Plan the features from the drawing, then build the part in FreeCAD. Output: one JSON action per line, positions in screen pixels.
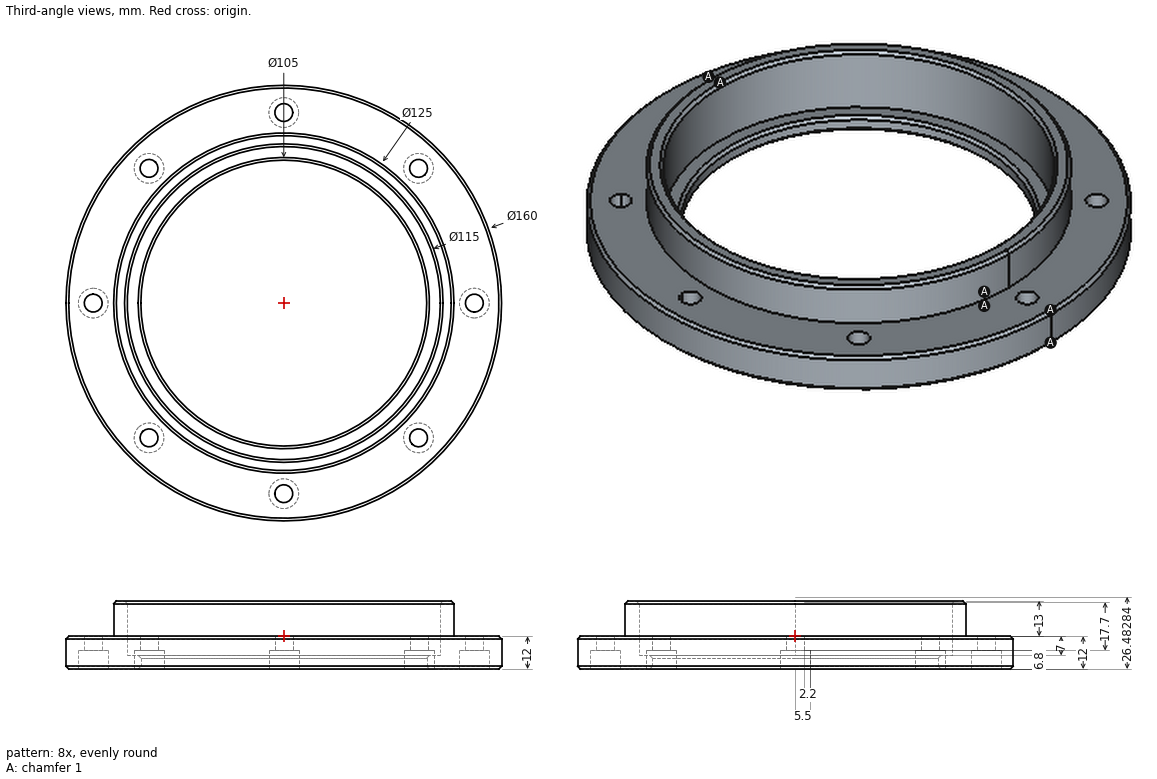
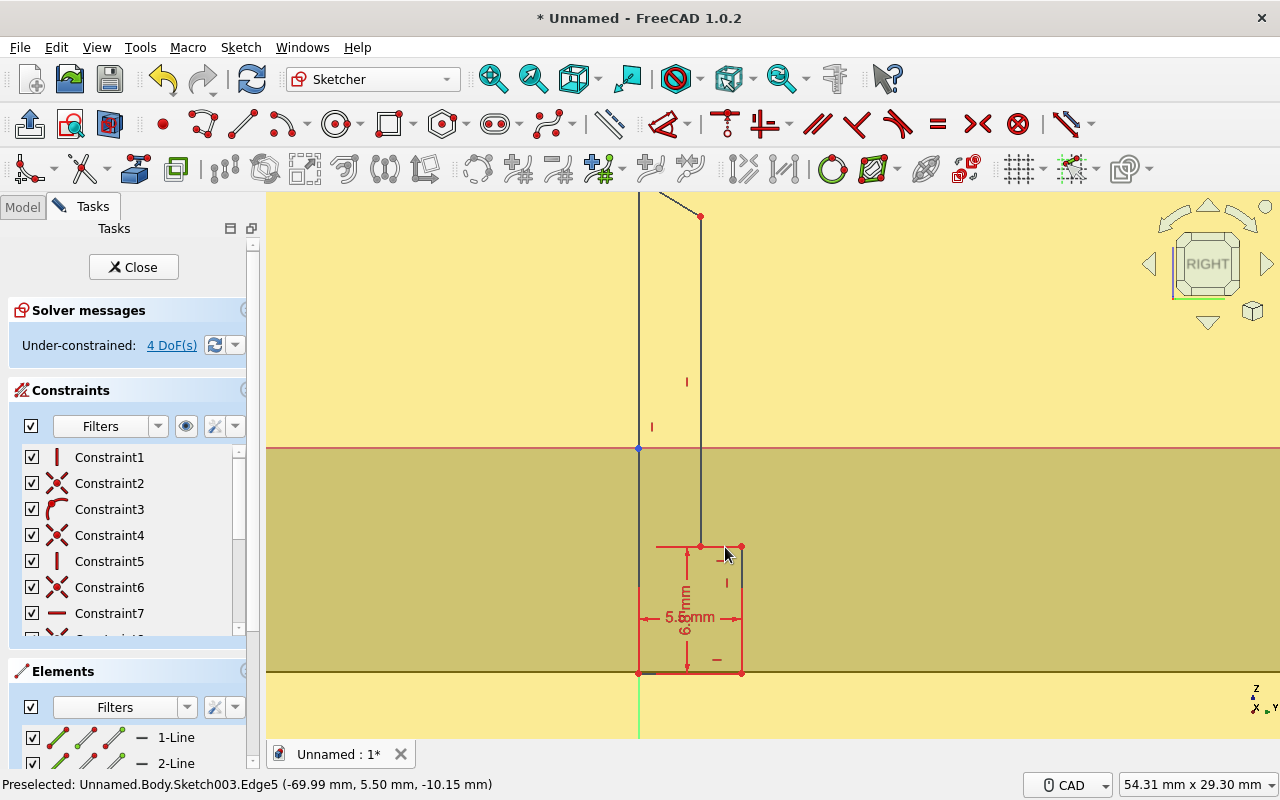
{"action": "left_click", "coordinate": [725, 547]}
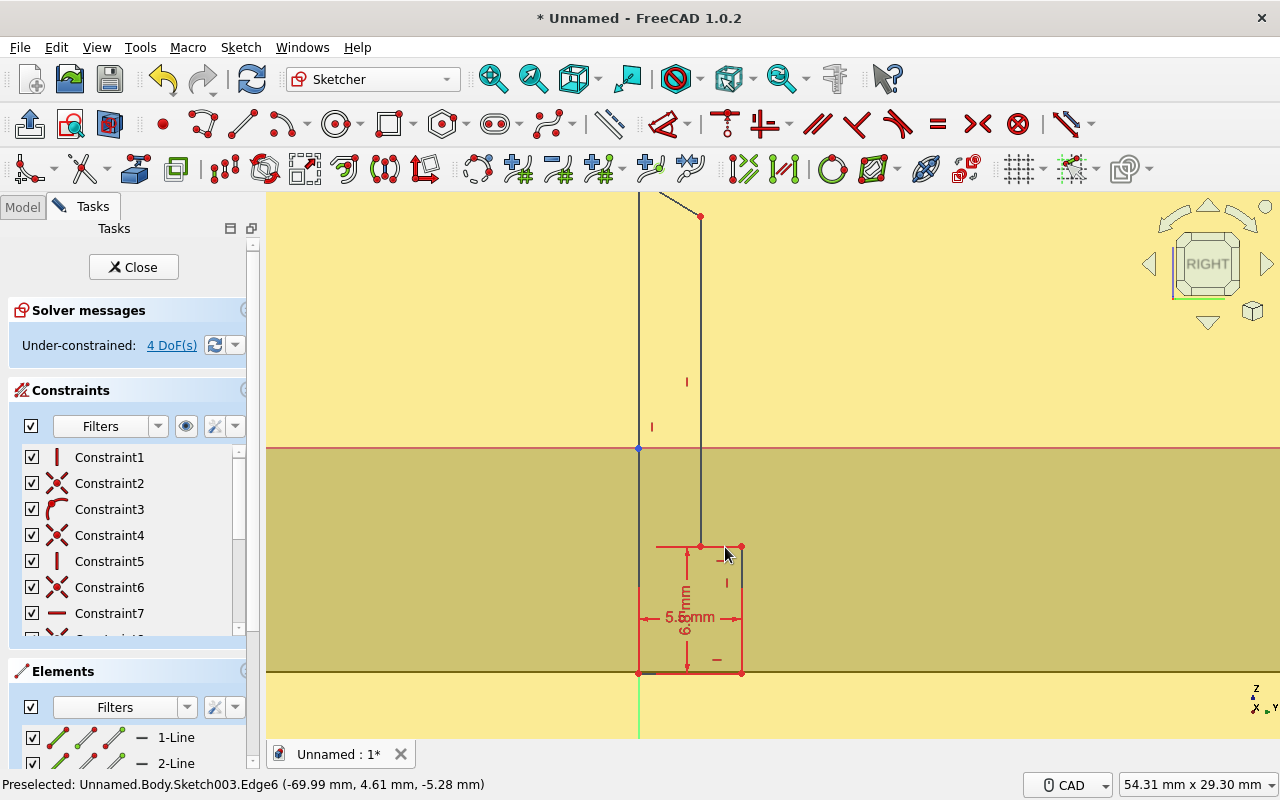
{"action": "key", "text": "l"}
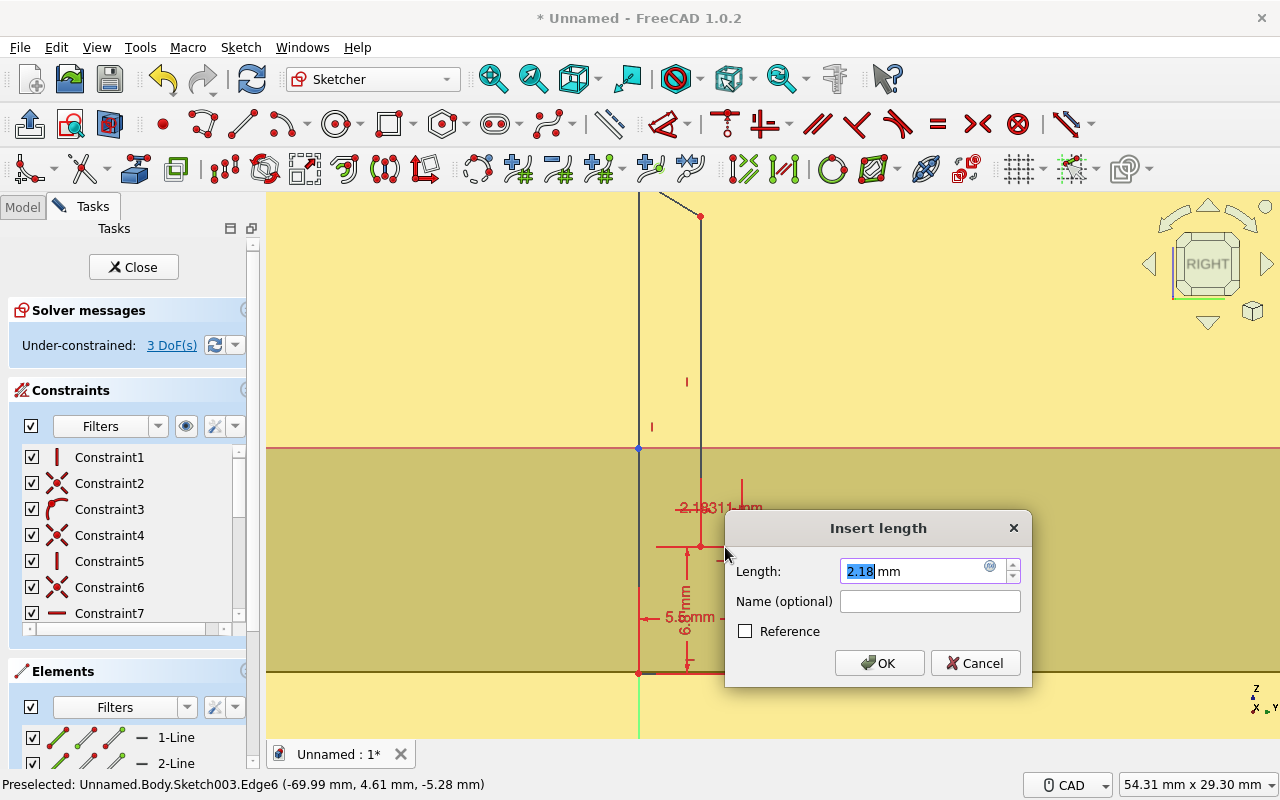
{"action": "type", "text": "2.2"}
{"action": "key", "text": "Return"}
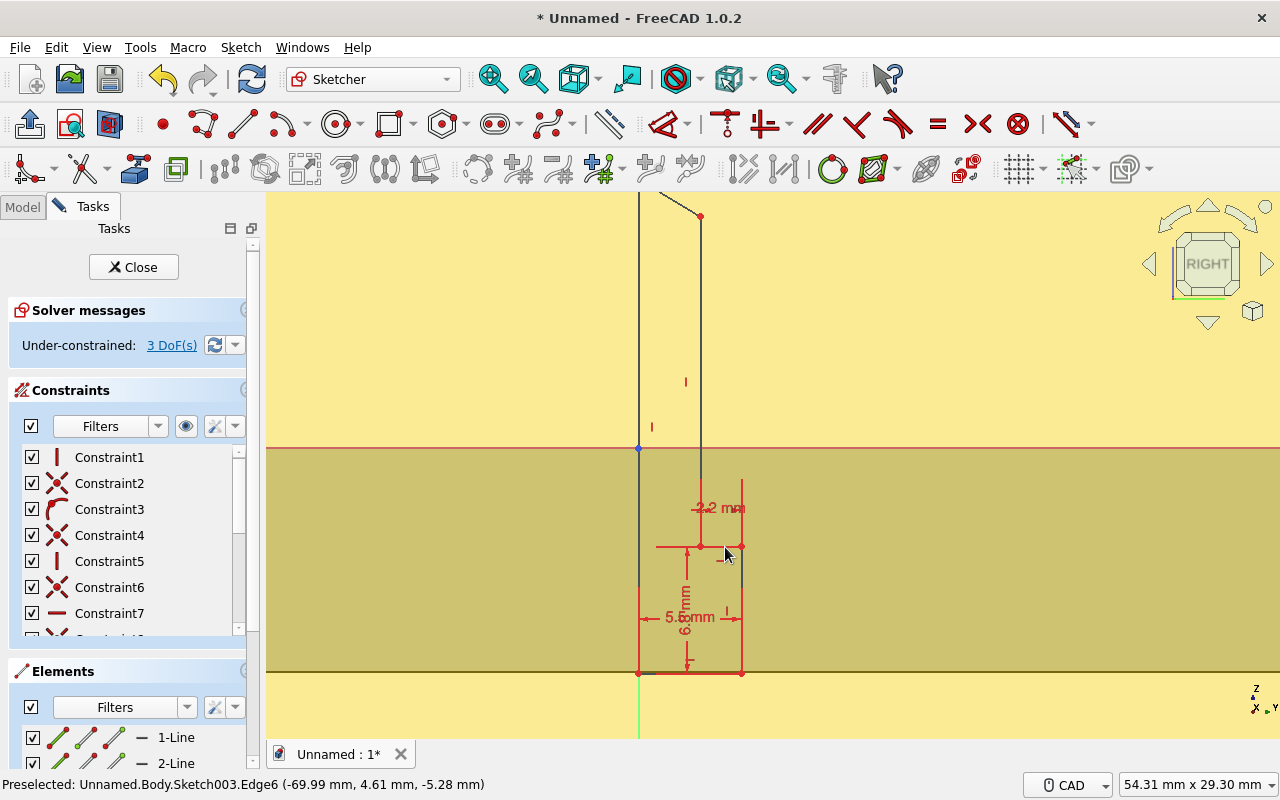
{"action": "left_click", "coordinate": [639, 674]}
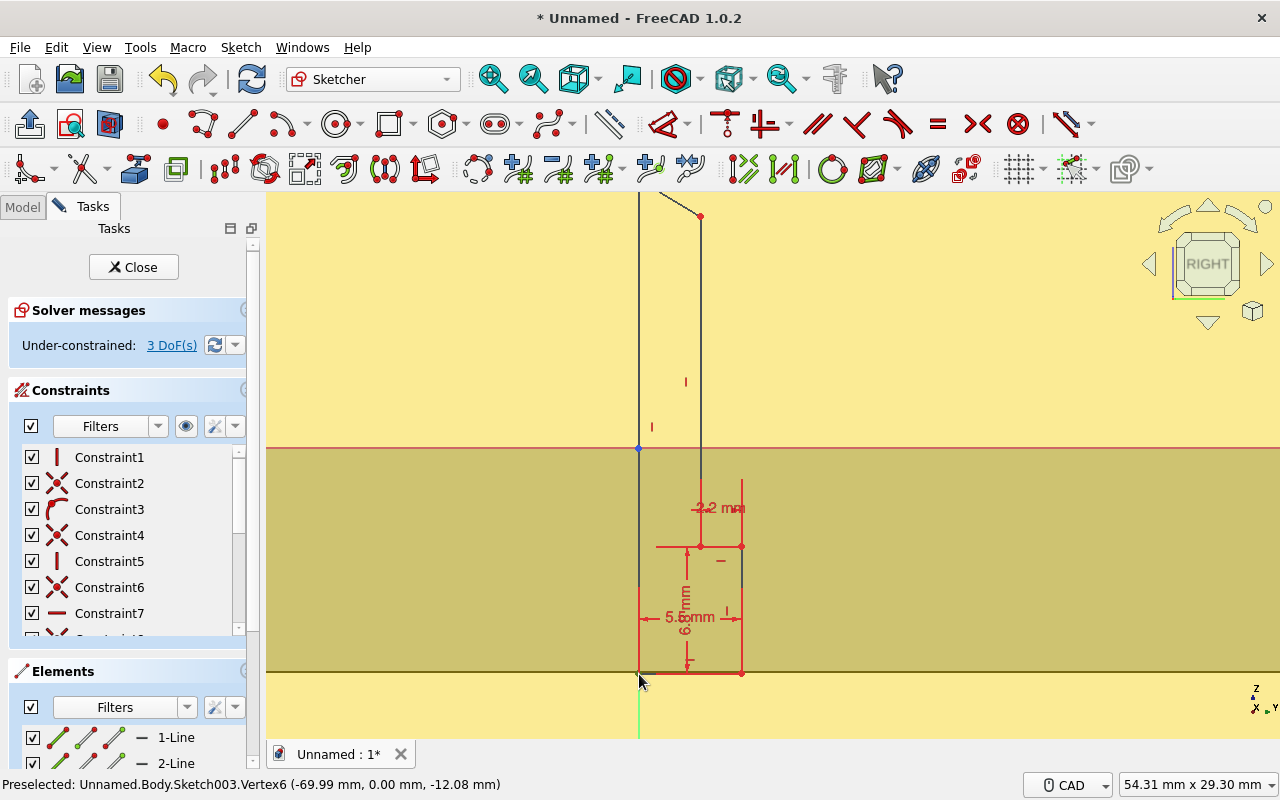
{"action": "key", "text": "i"}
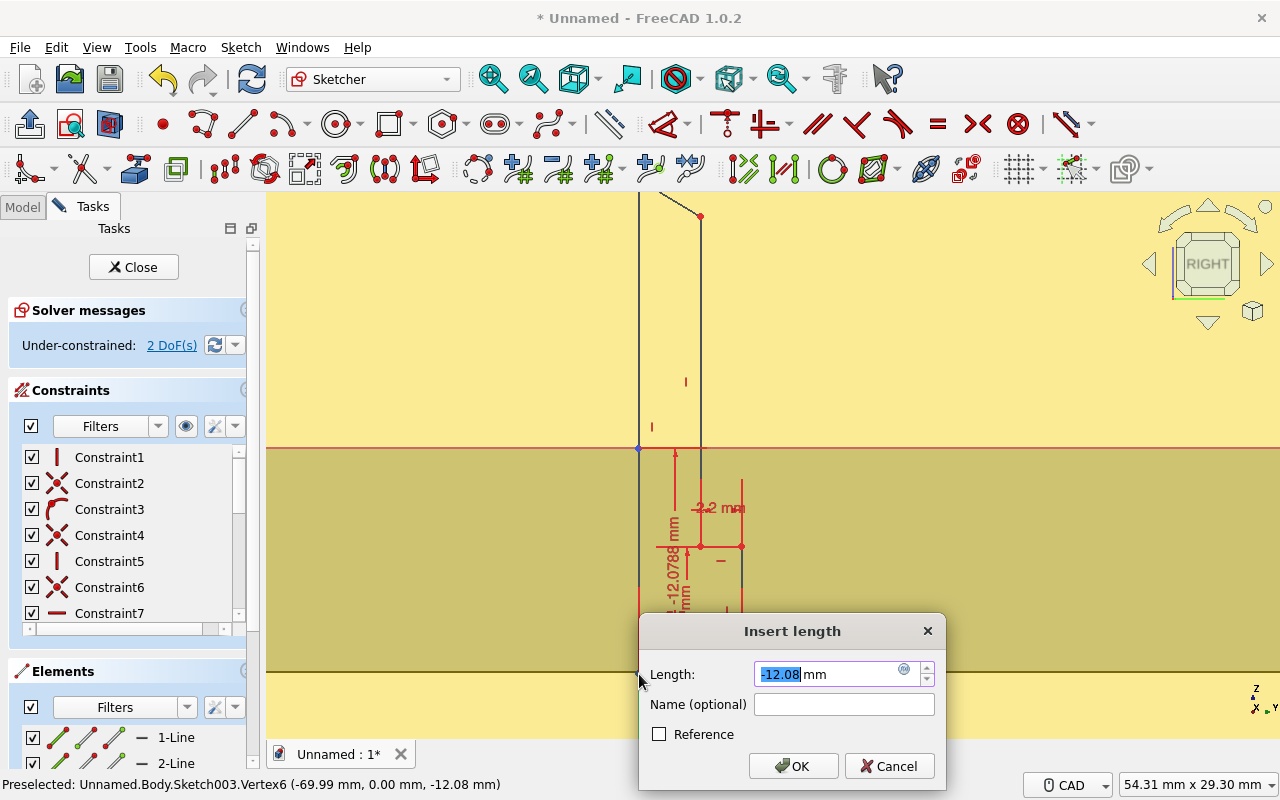
{"action": "type", "text": "-12"}
{"action": "key", "text": "Return"}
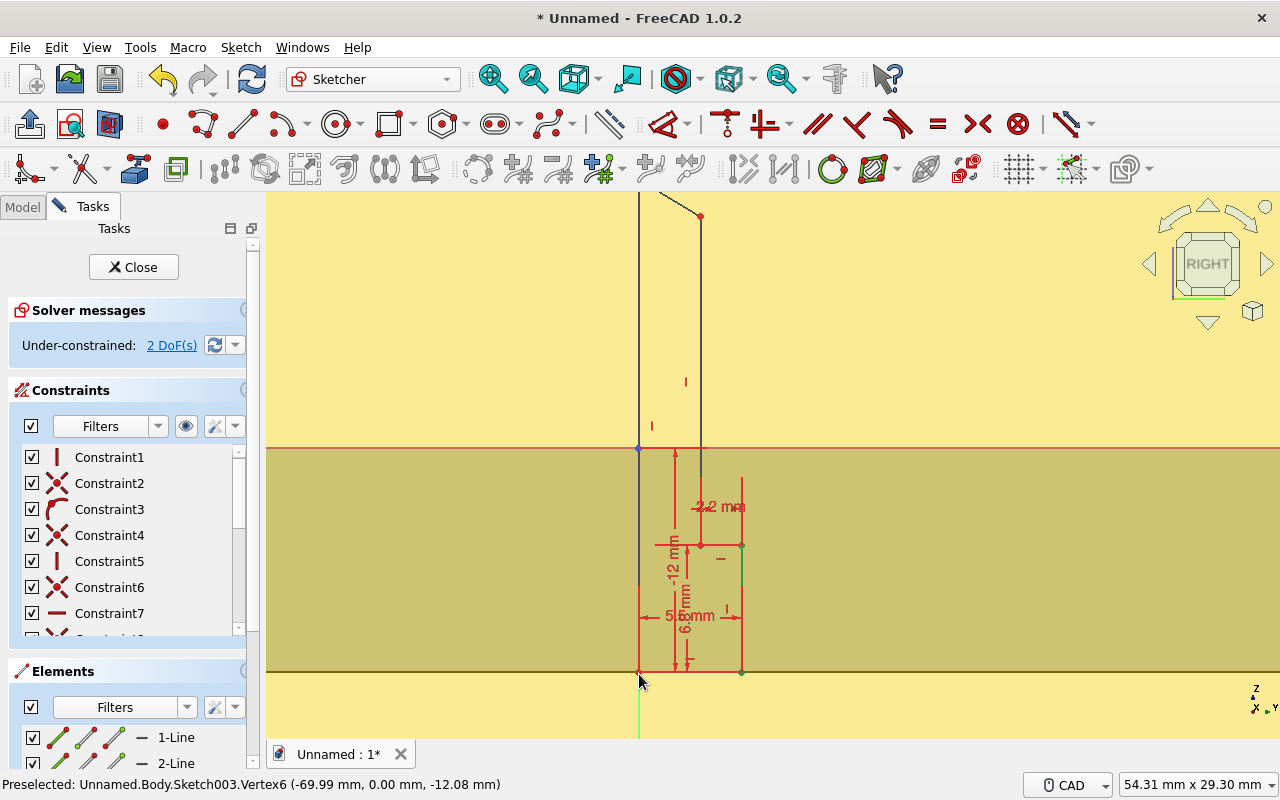
{"action": "left_click", "coordinate": [701, 447]}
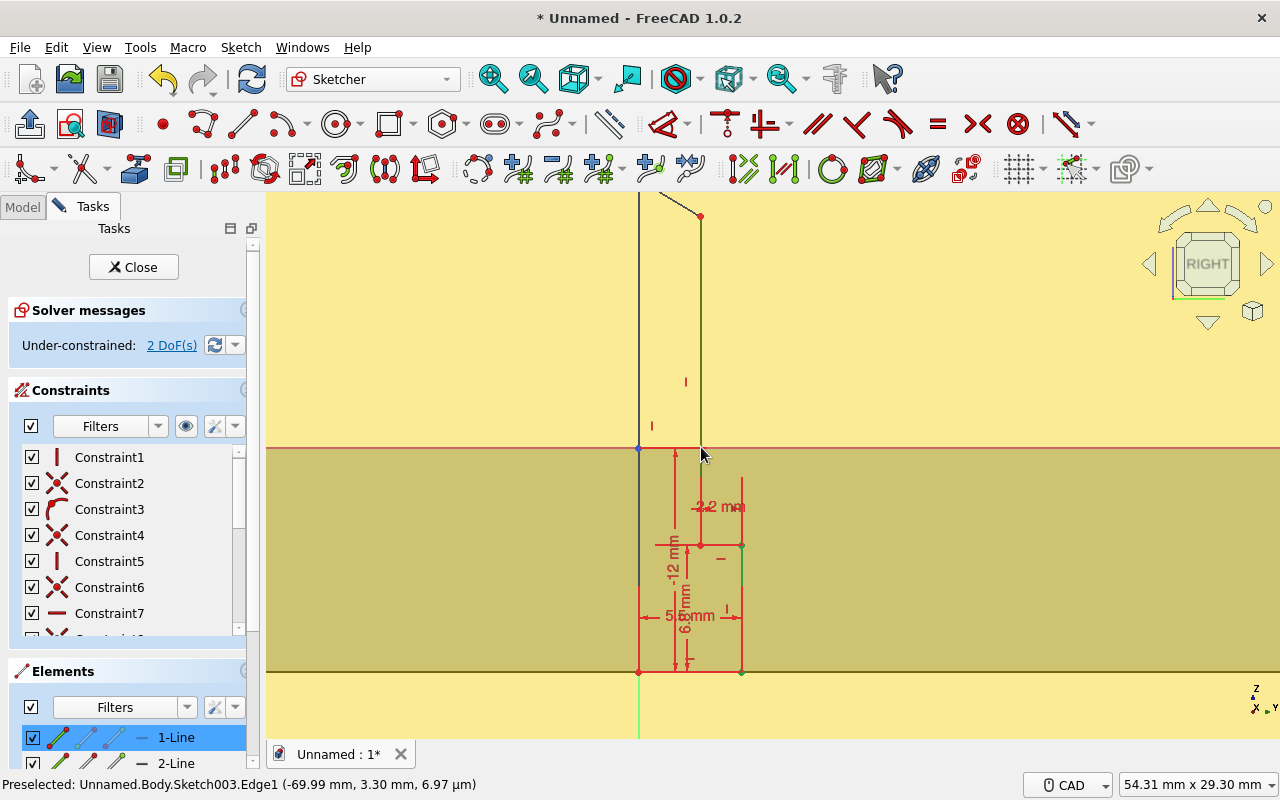
{"action": "key", "text": "i"}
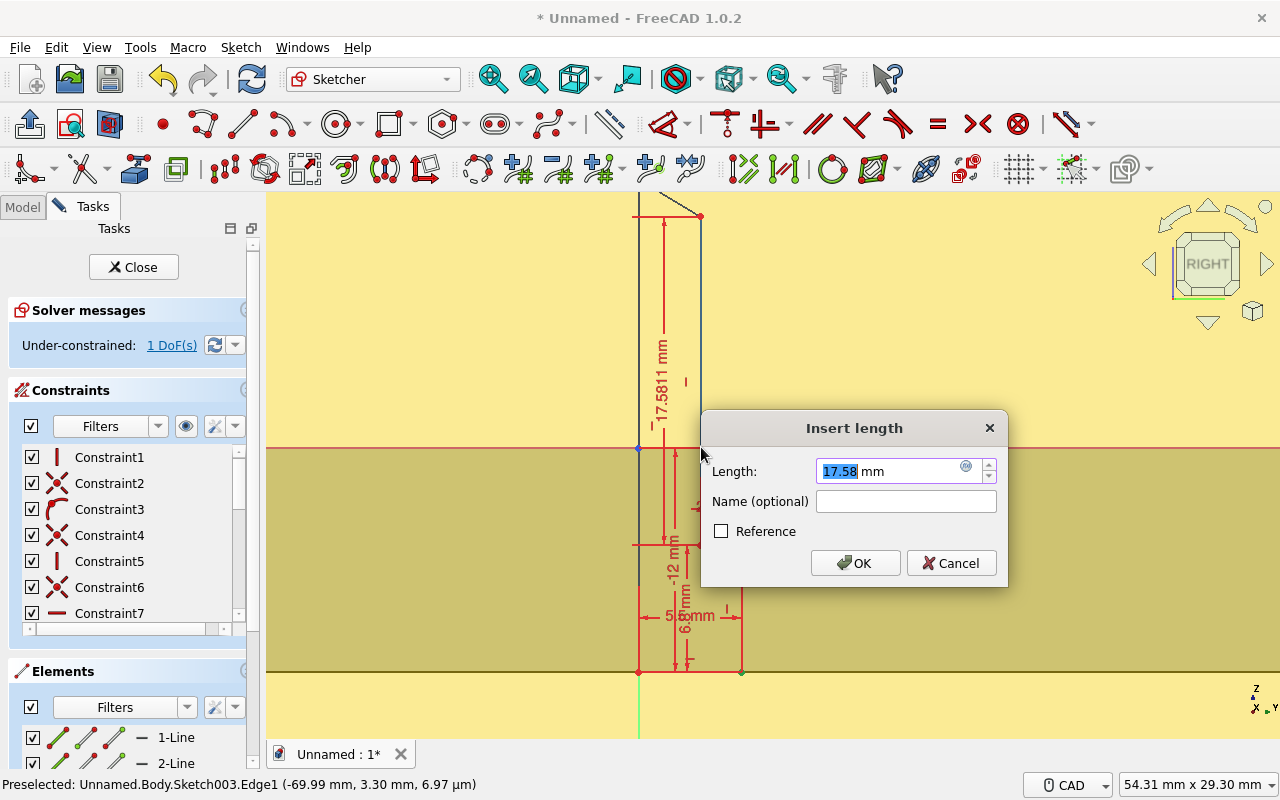
{"action": "type", "text": "17.7"}
{"action": "key", "text": "Return"}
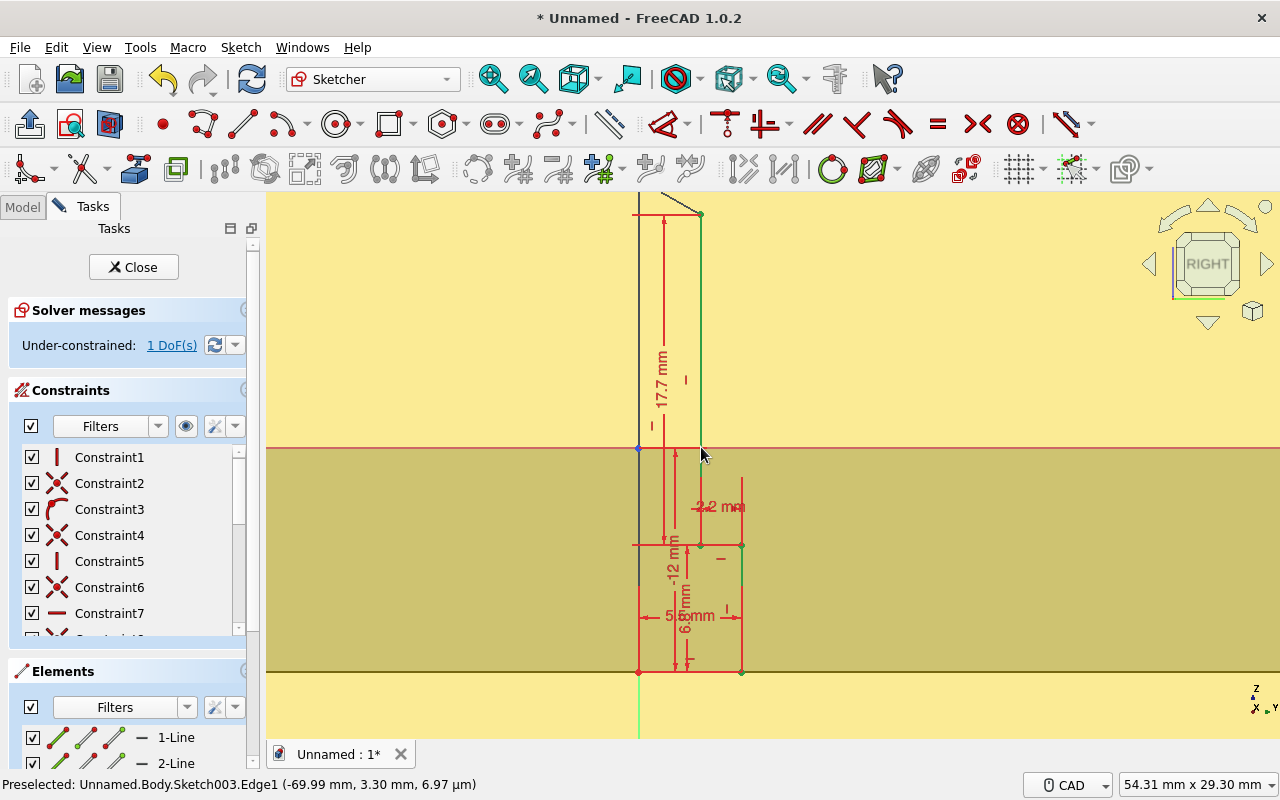
{"action": "left_click", "coordinate": [639, 327]}